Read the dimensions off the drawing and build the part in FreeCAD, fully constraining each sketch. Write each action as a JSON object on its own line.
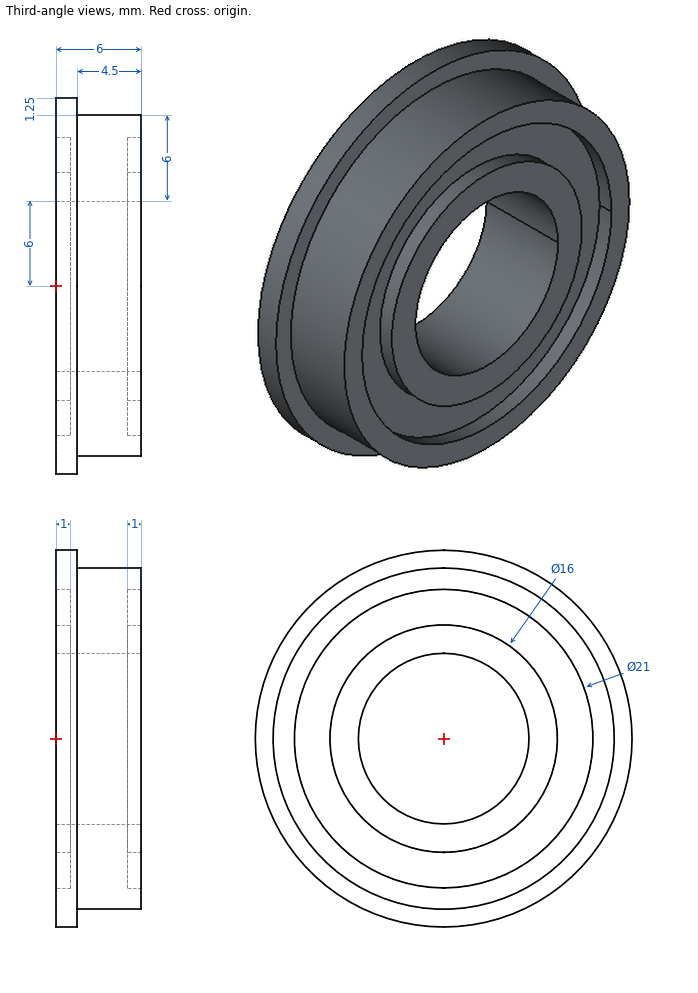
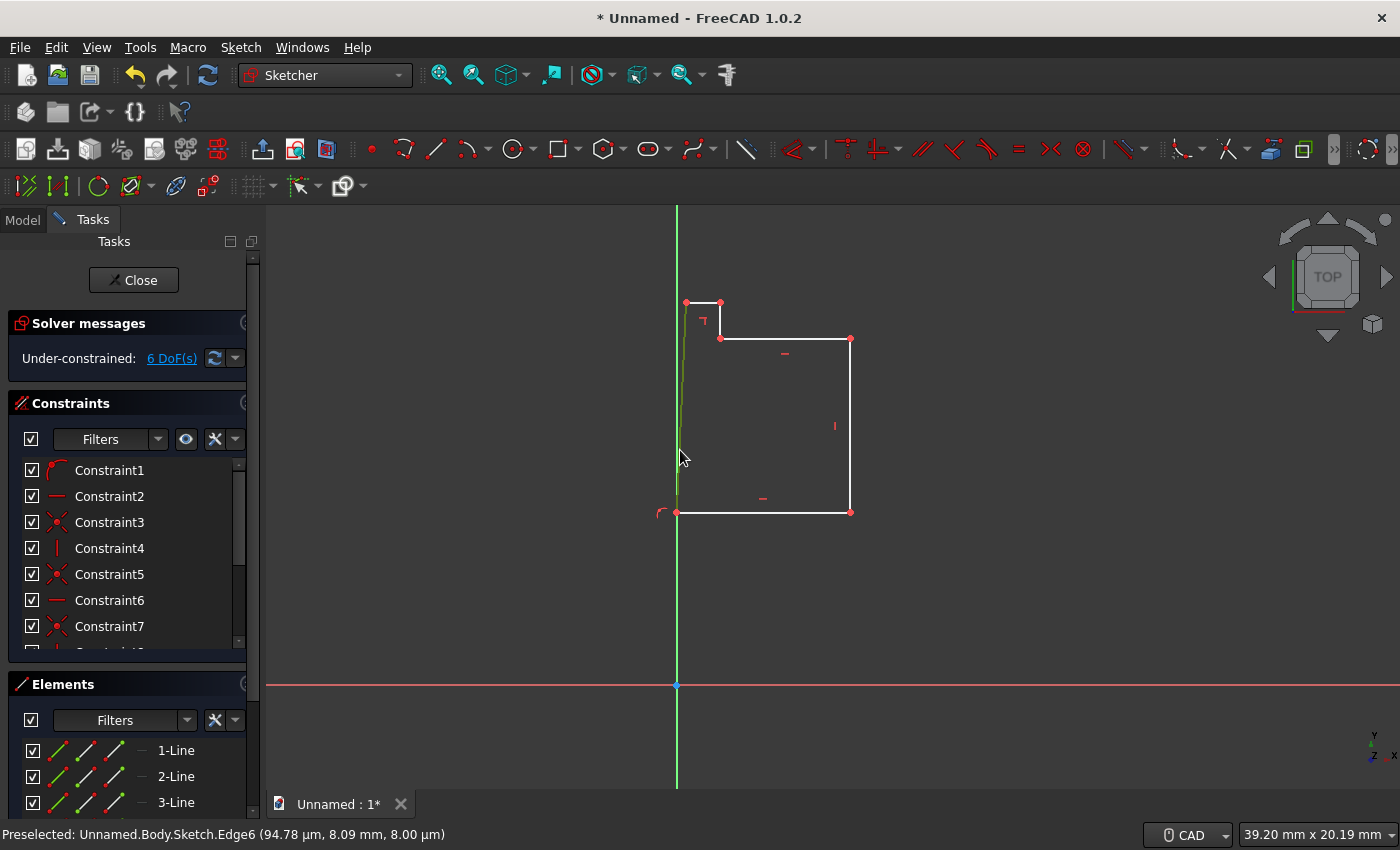
{"action": "left_click", "coordinate": [900, 150]}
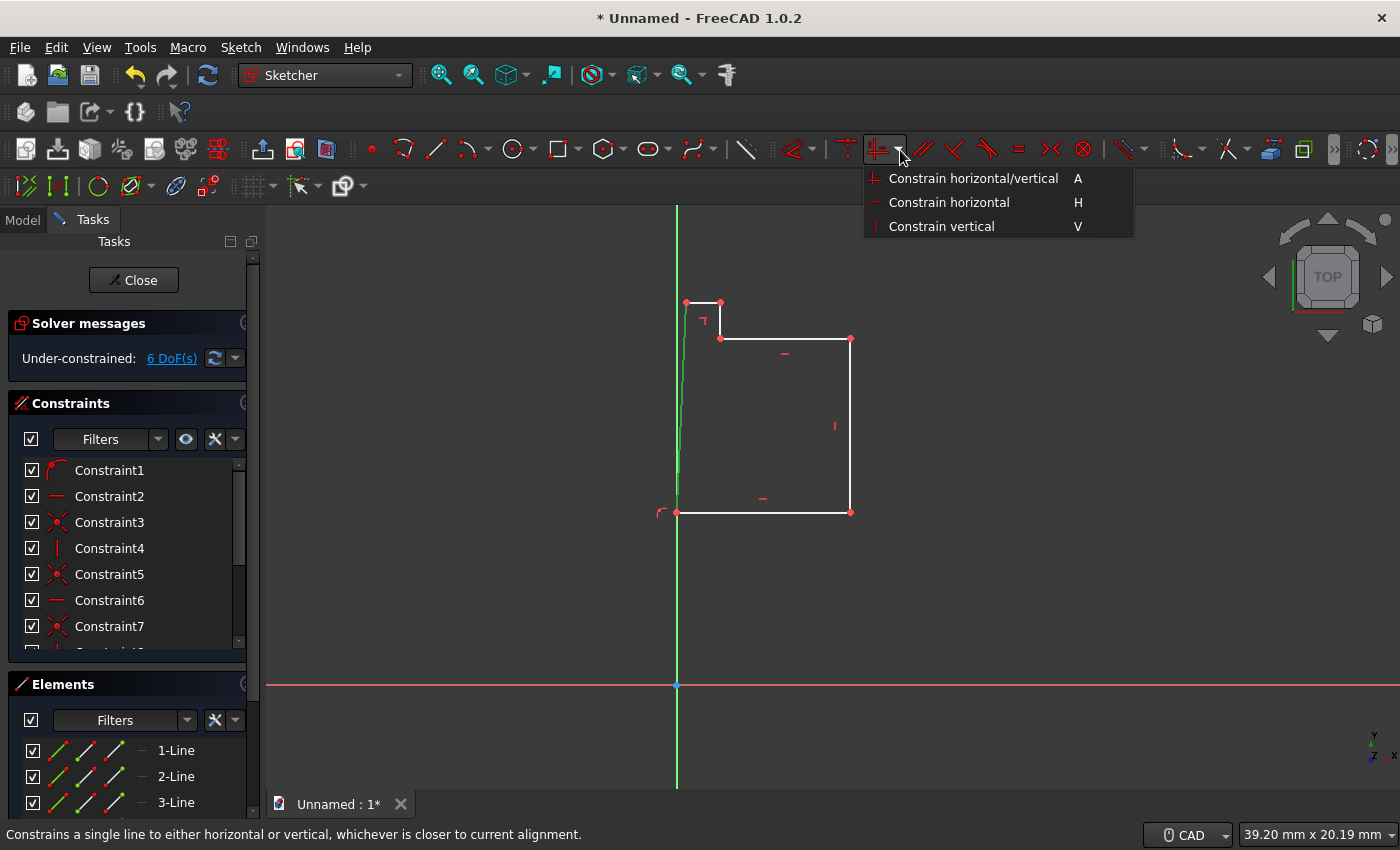
{"action": "left_click", "coordinate": [999, 226]}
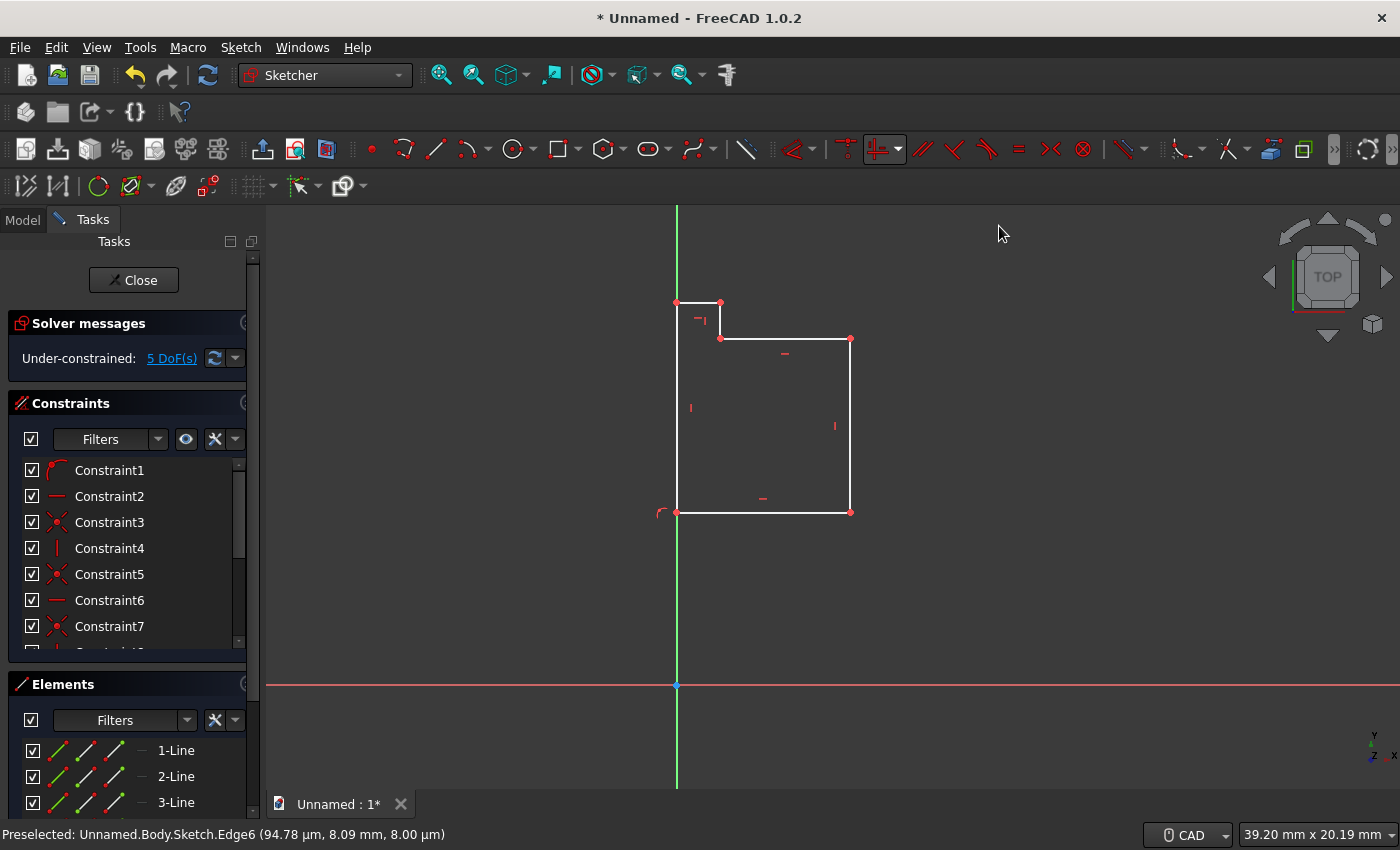
{"action": "left_click", "coordinate": [792, 150]}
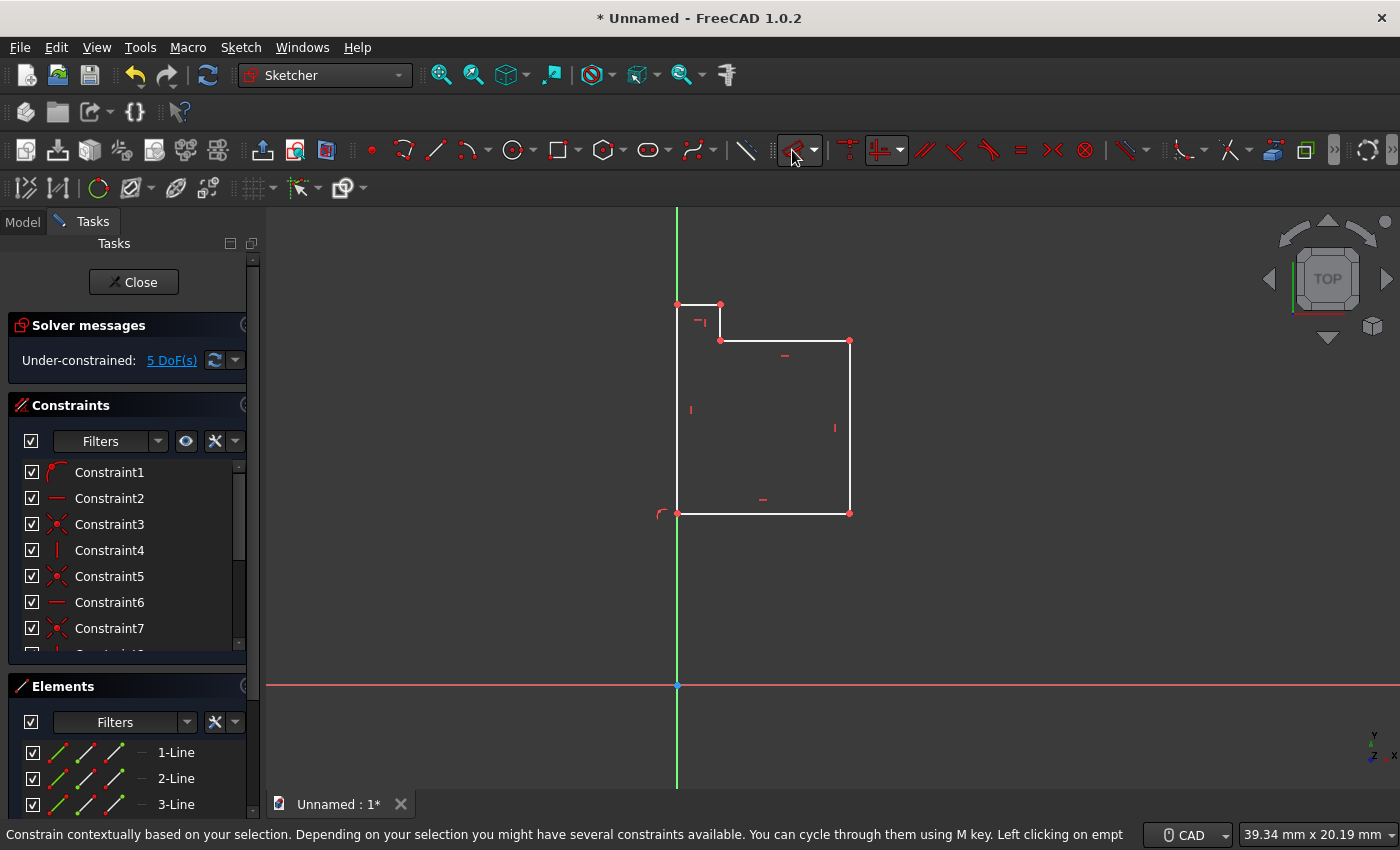
{"action": "left_click", "coordinate": [729, 514]}
{"action": "left_click", "coordinate": [764, 548]}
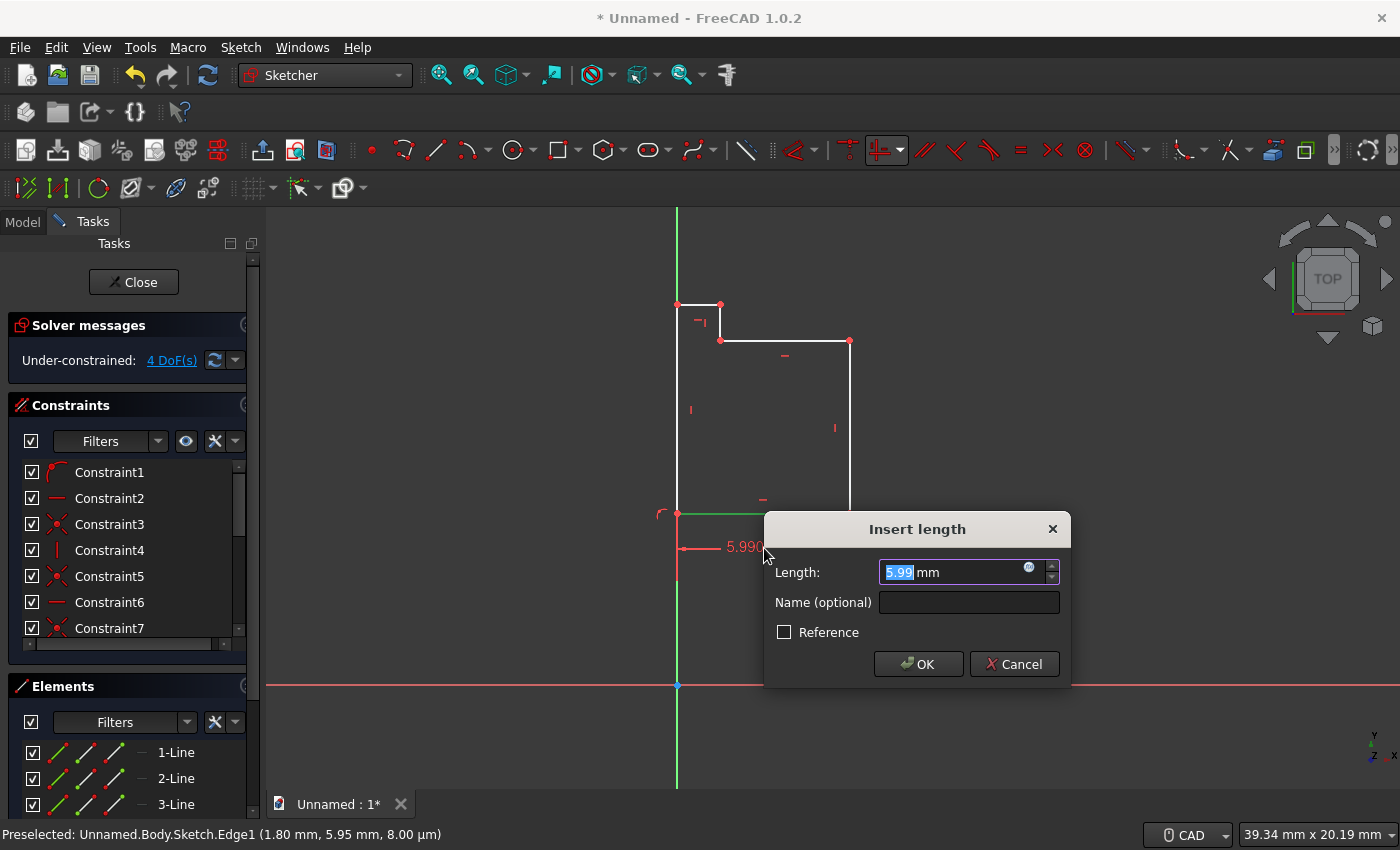
{"action": "type", "text": "6"}
{"action": "key", "text": "Return"}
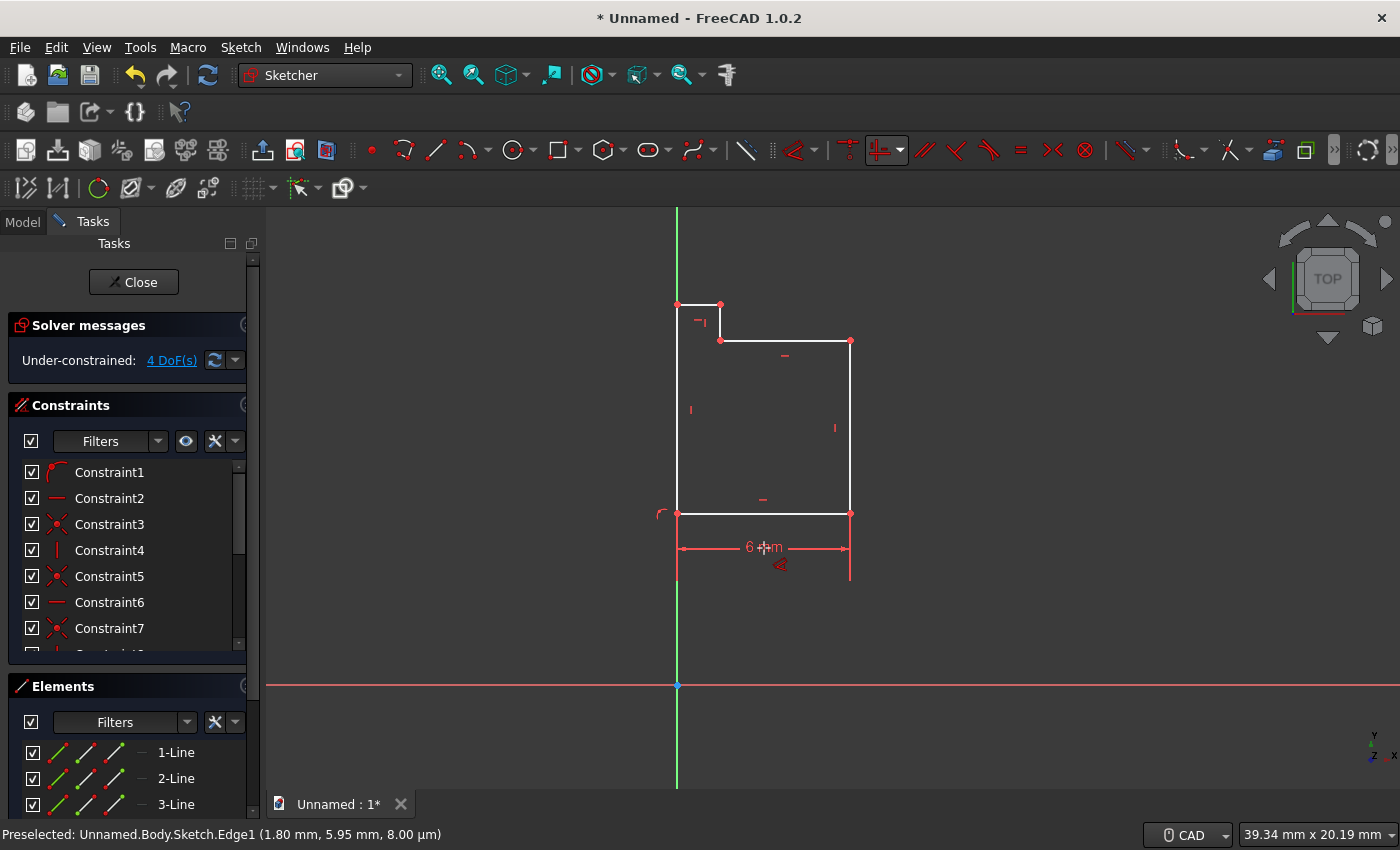
{"action": "left_click", "coordinate": [850, 462]}
{"action": "left_click", "coordinate": [884, 427]}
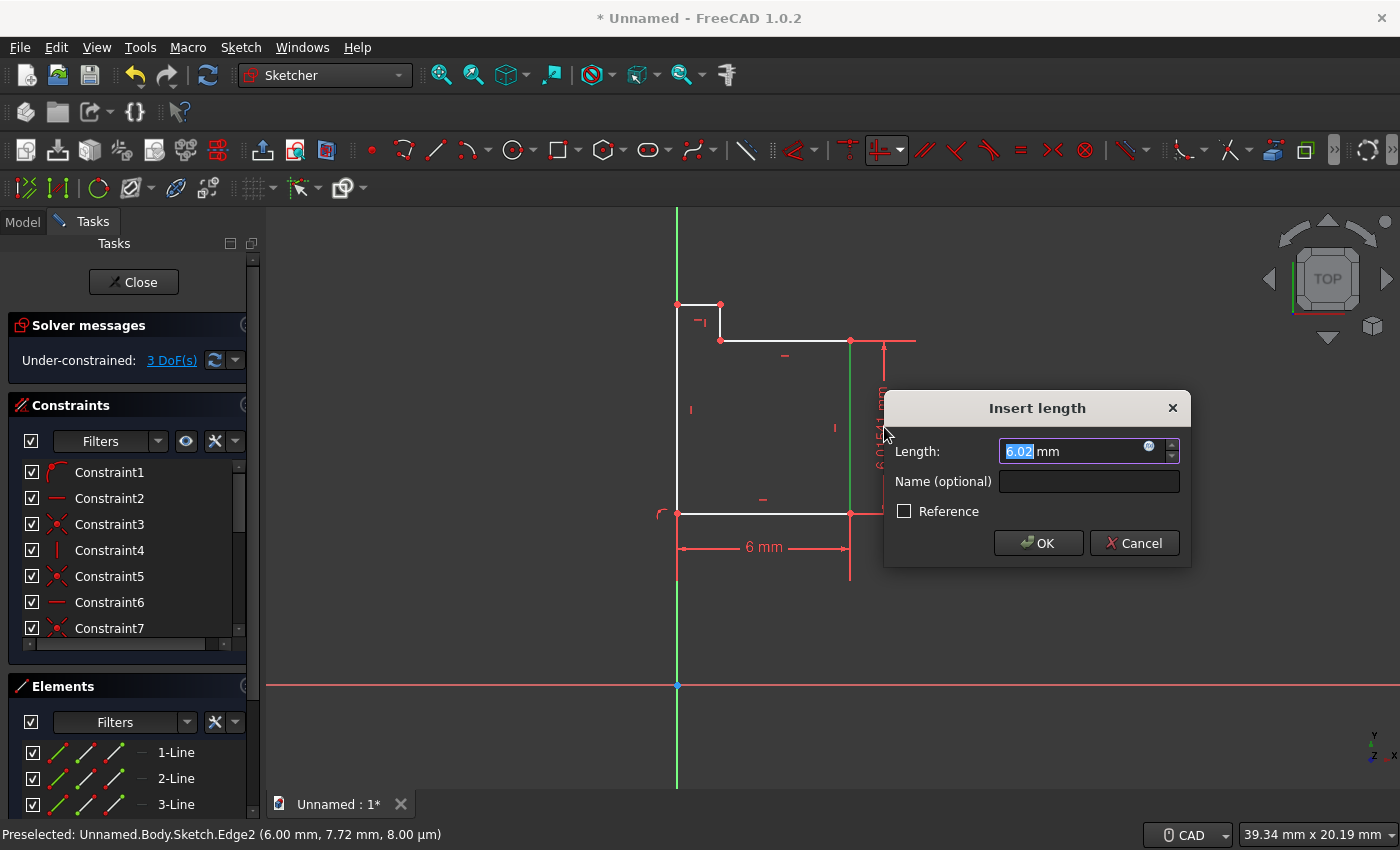
{"action": "type", "text": "6"}
{"action": "key", "text": "Return"}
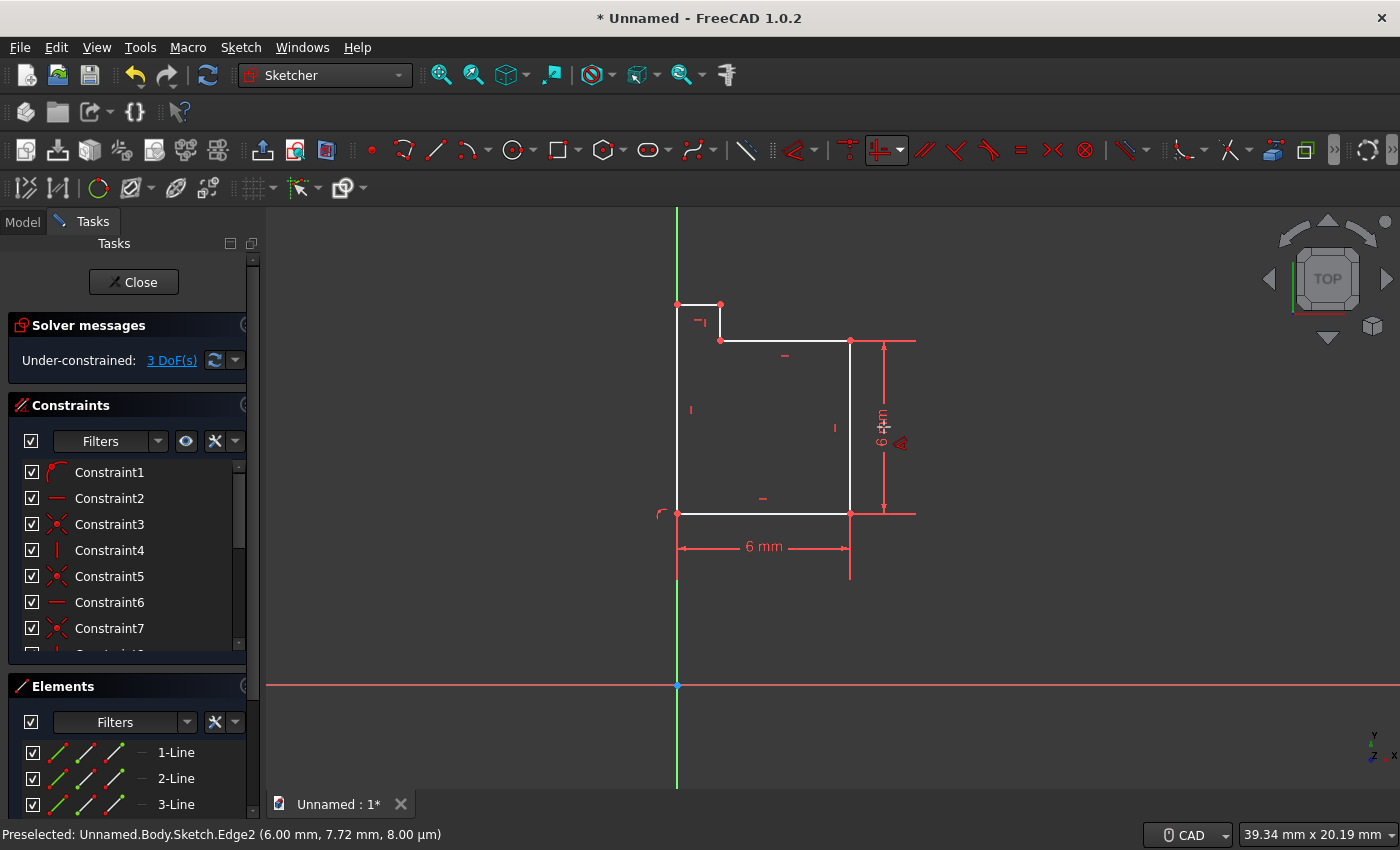
{"action": "left_click", "coordinate": [677, 514]}
{"action": "left_click", "coordinate": [643, 599]}